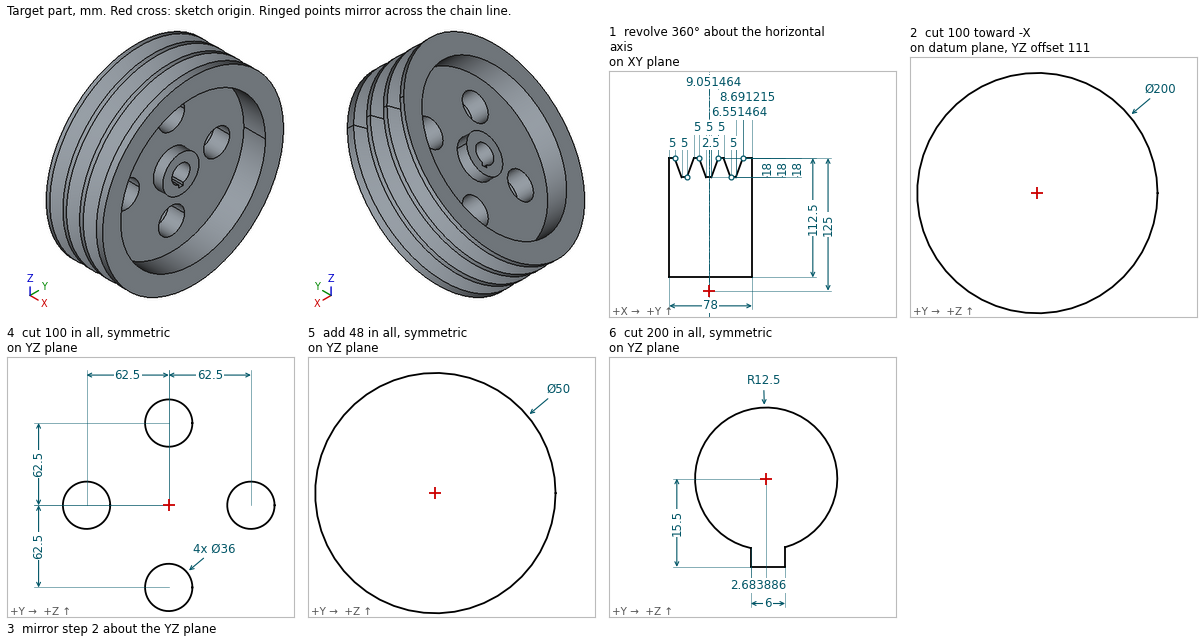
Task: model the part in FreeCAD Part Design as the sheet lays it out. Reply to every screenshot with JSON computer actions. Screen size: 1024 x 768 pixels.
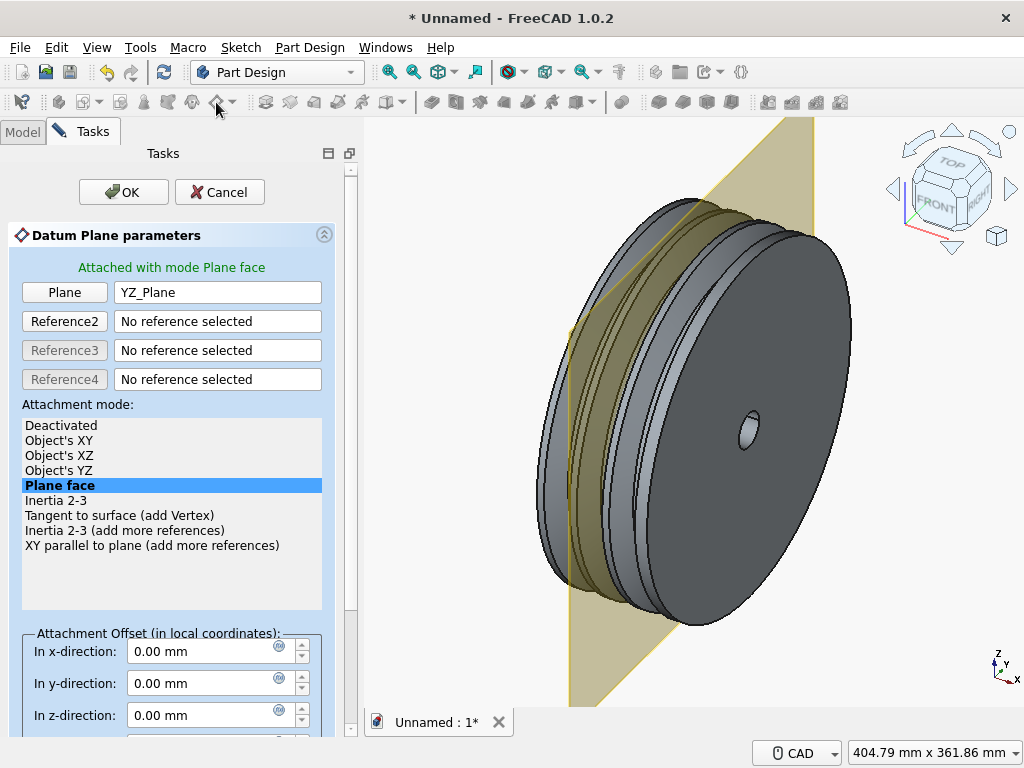
{"action": "triple_click", "coordinate": [210, 715]}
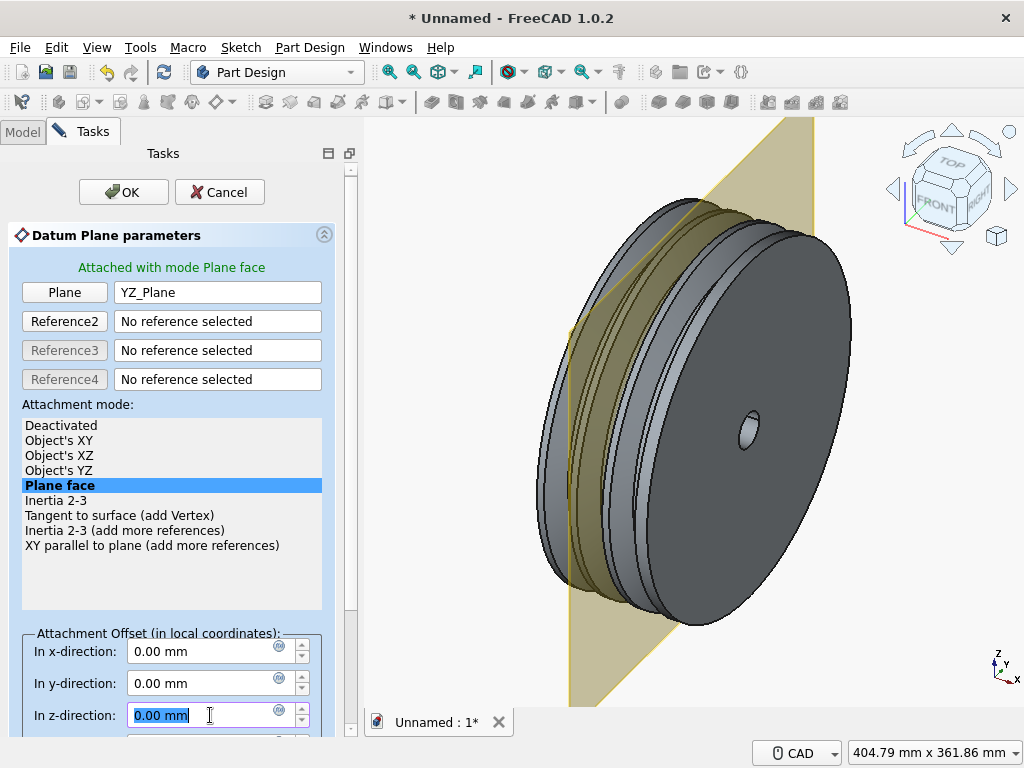
{"action": "type", "text": "111"}
{"action": "key", "text": "Tab"}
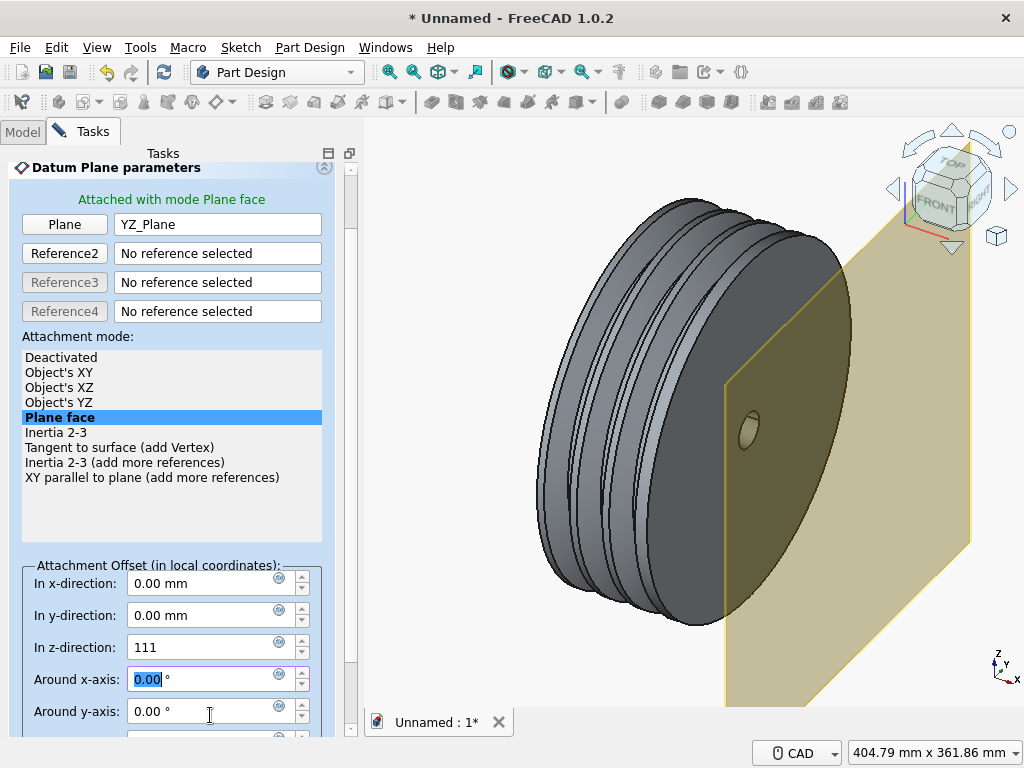
{"action": "scroll", "coordinate": [351, 450], "scroll_direction": "up", "scroll_amount": 2}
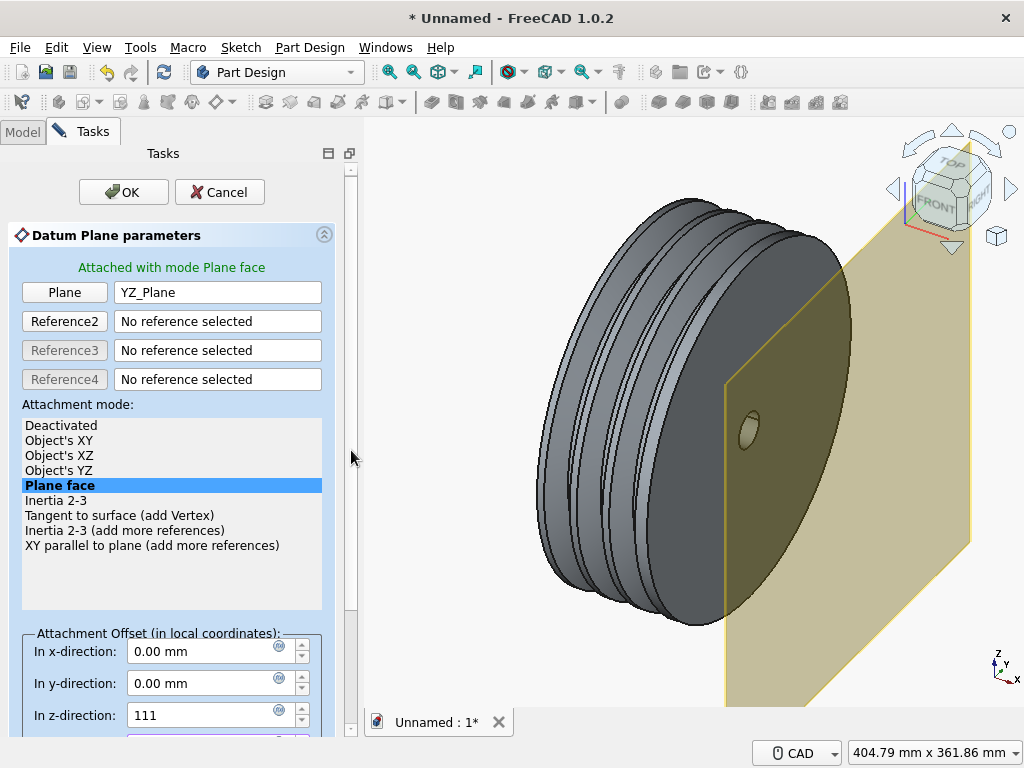
{"action": "left_click", "coordinate": [124, 192]}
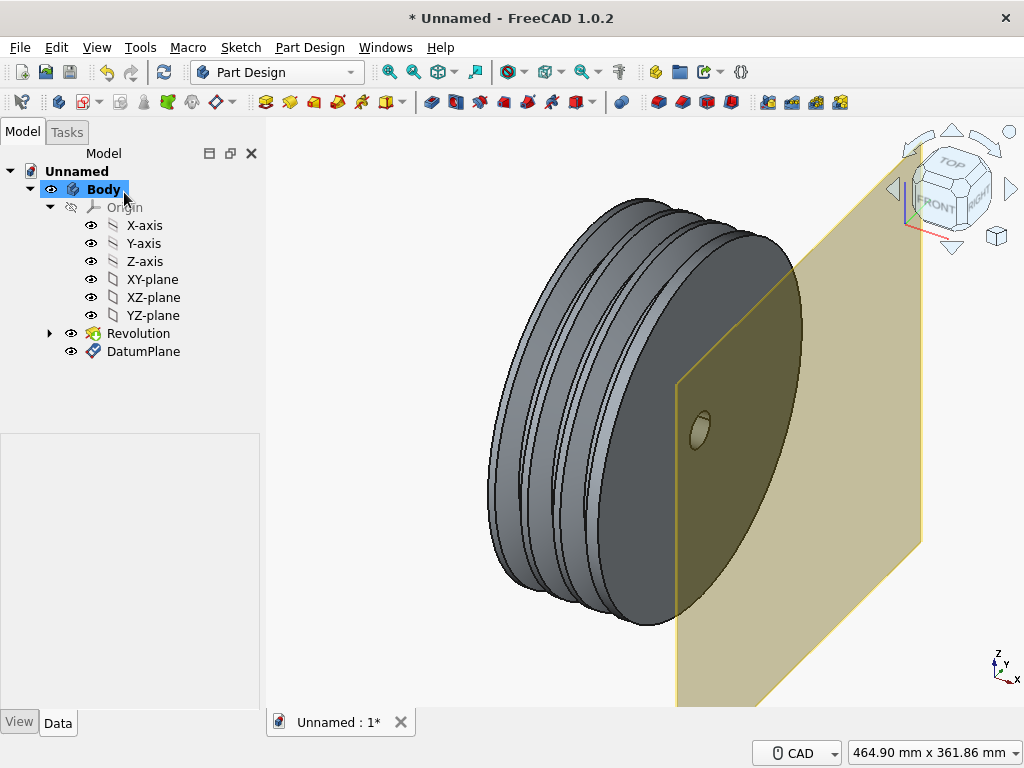
{"action": "left_click", "coordinate": [116, 351]}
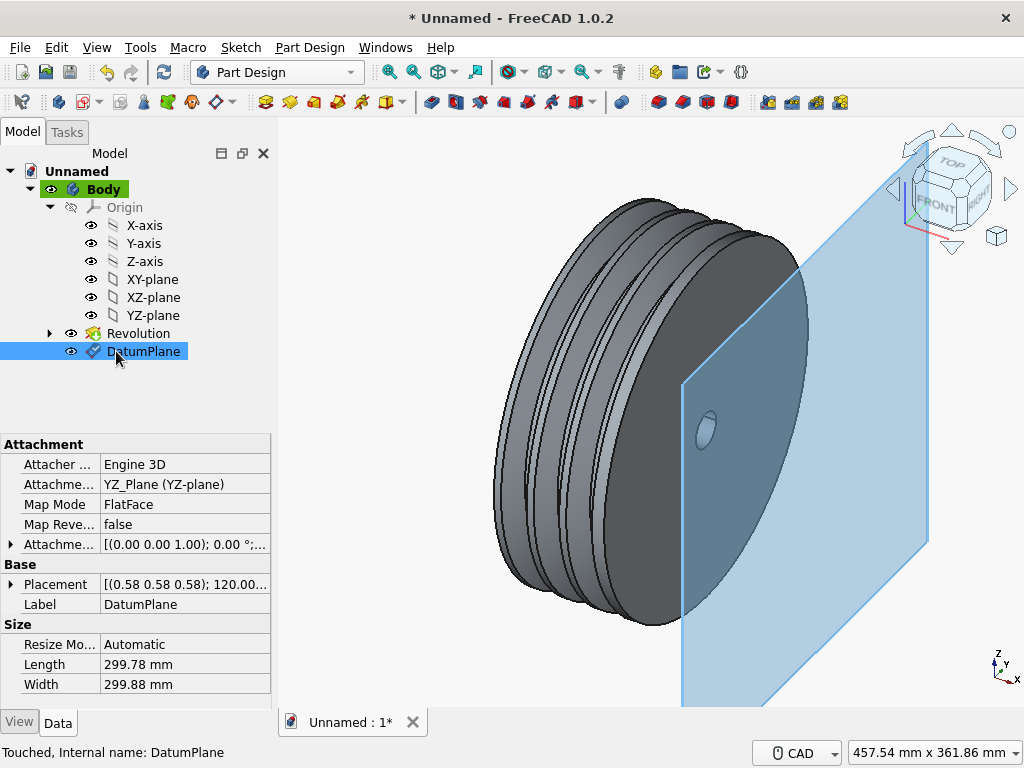
{"action": "left_click", "coordinate": [84, 102]}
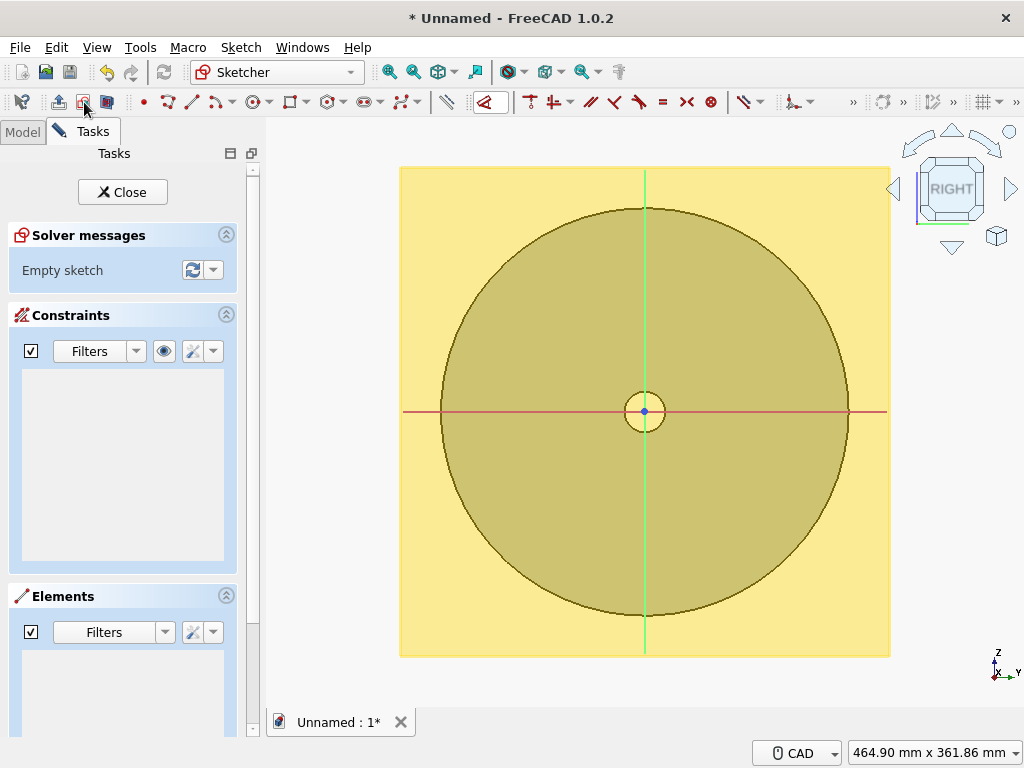
{"action": "left_click", "coordinate": [254, 102]}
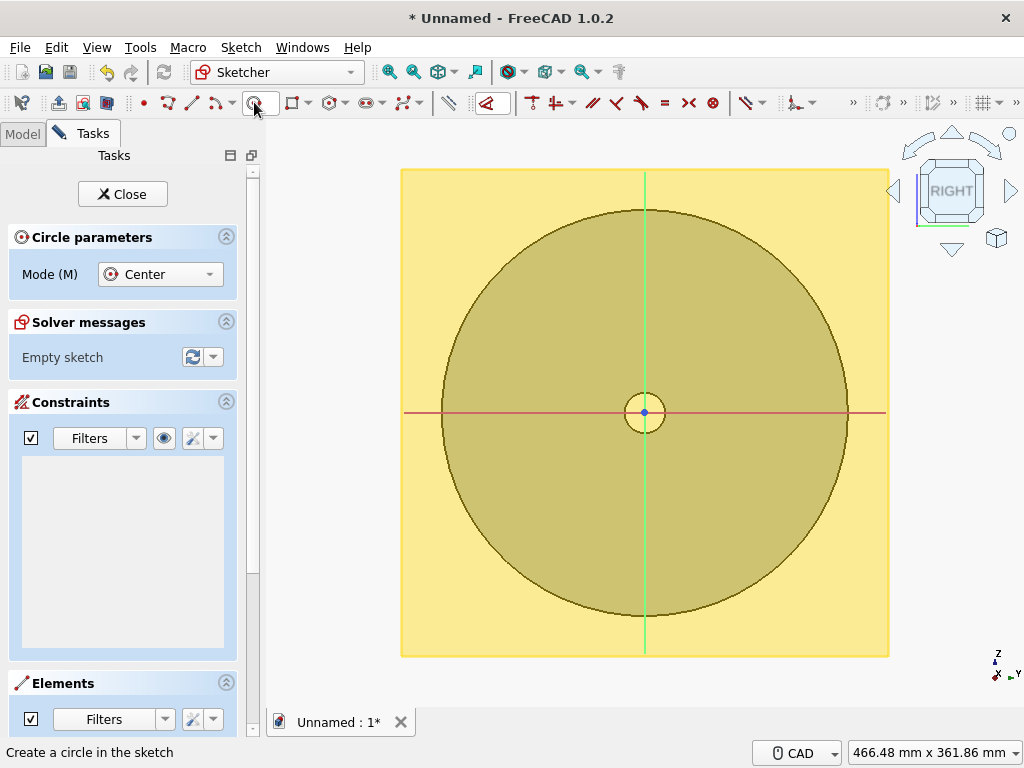
{"action": "left_click", "coordinate": [645, 413]}
{"action": "left_click", "coordinate": [760, 298]}
{"action": "key", "text": "Escape"}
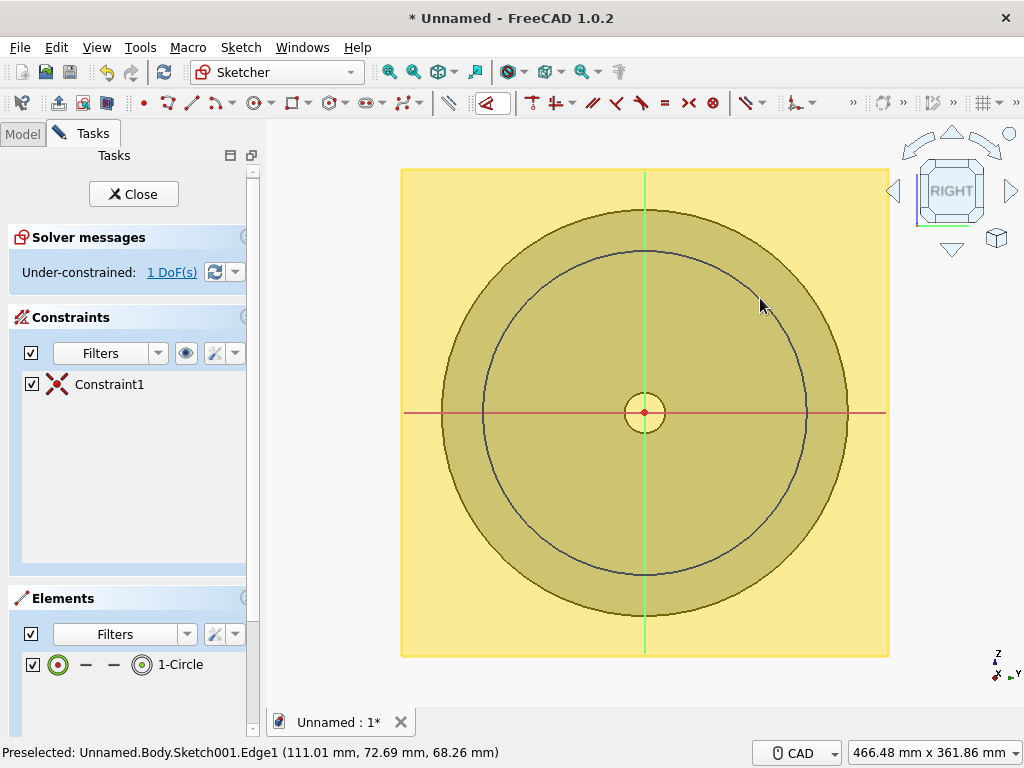
{"action": "left_click", "coordinate": [759, 298]}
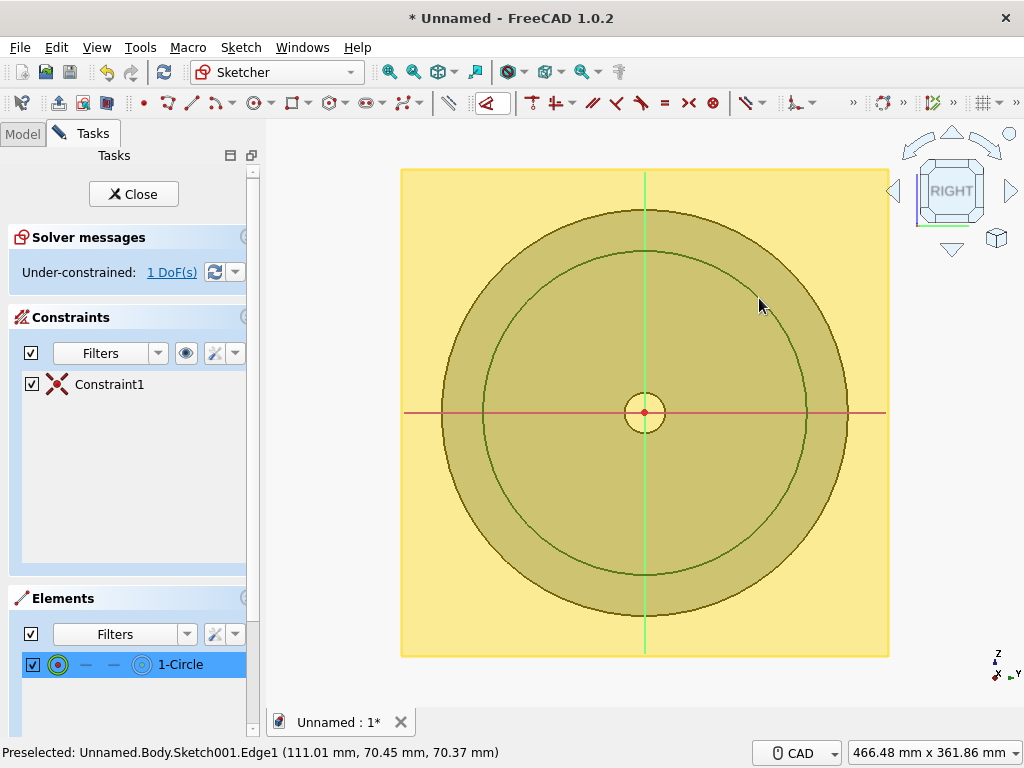
{"action": "left_click", "coordinate": [504, 104]}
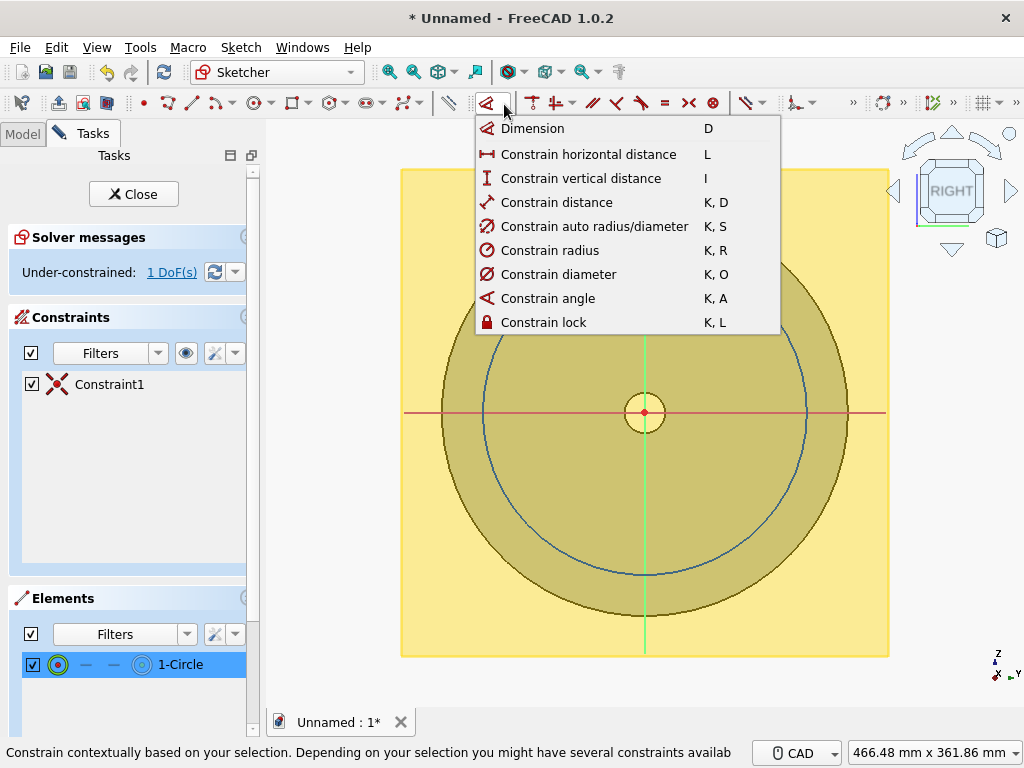
{"action": "left_click", "coordinate": [628, 274]}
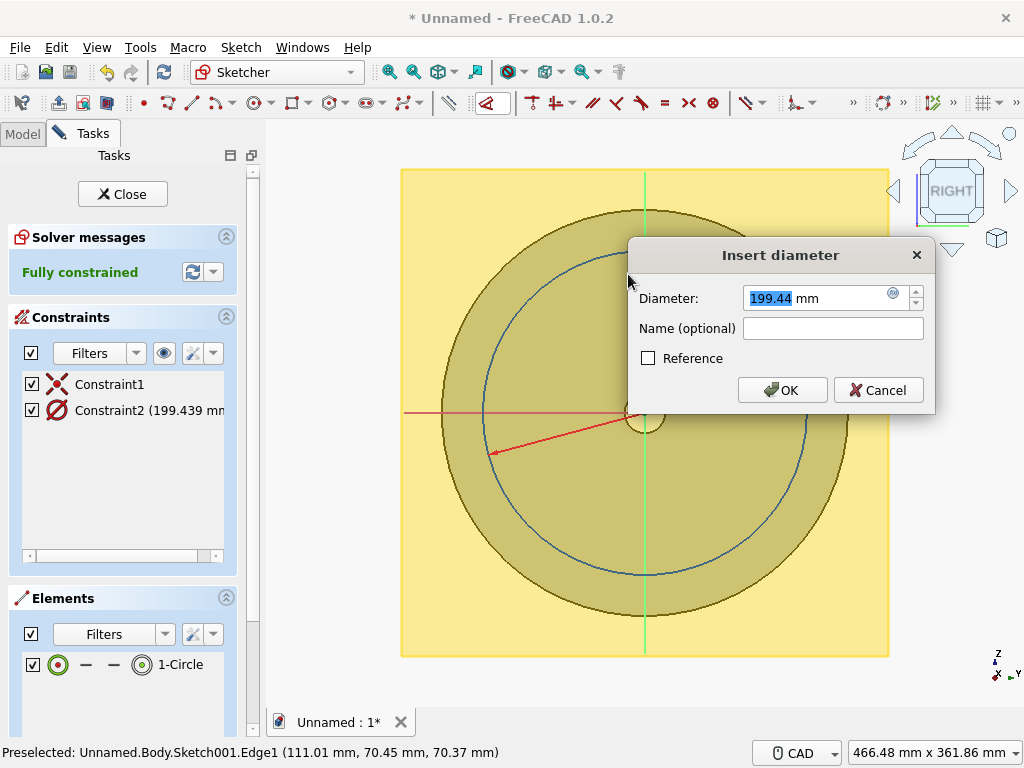
{"action": "type", "text": "200"}
{"action": "key", "text": "Return"}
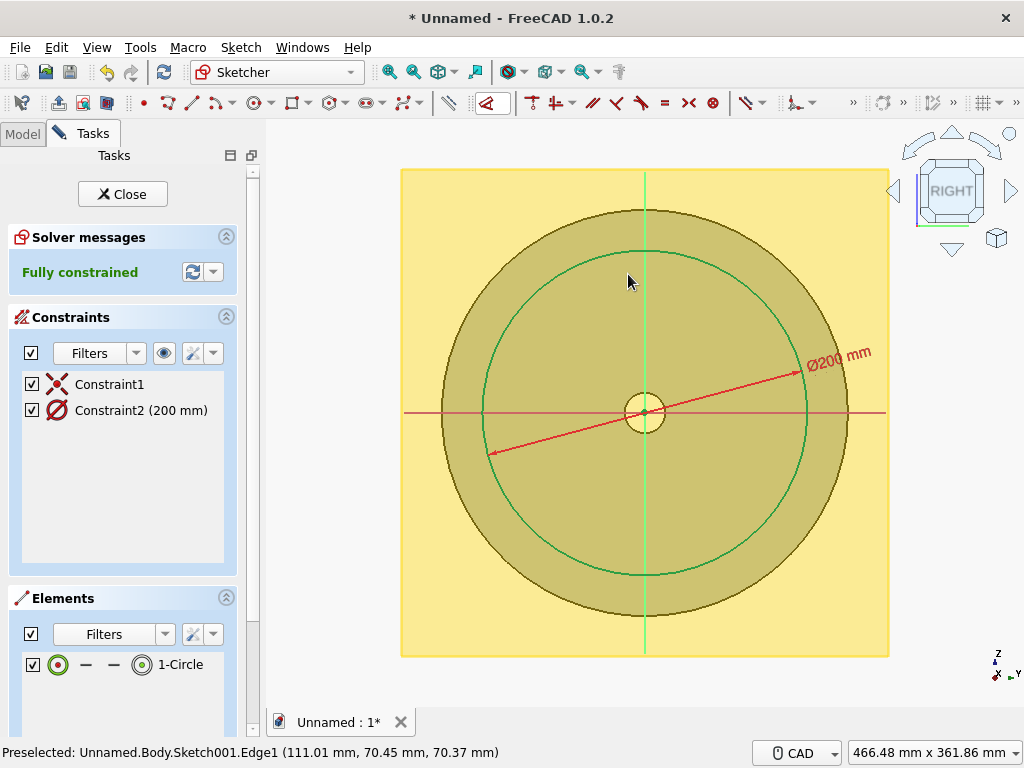
{"action": "left_click", "coordinate": [123, 194]}